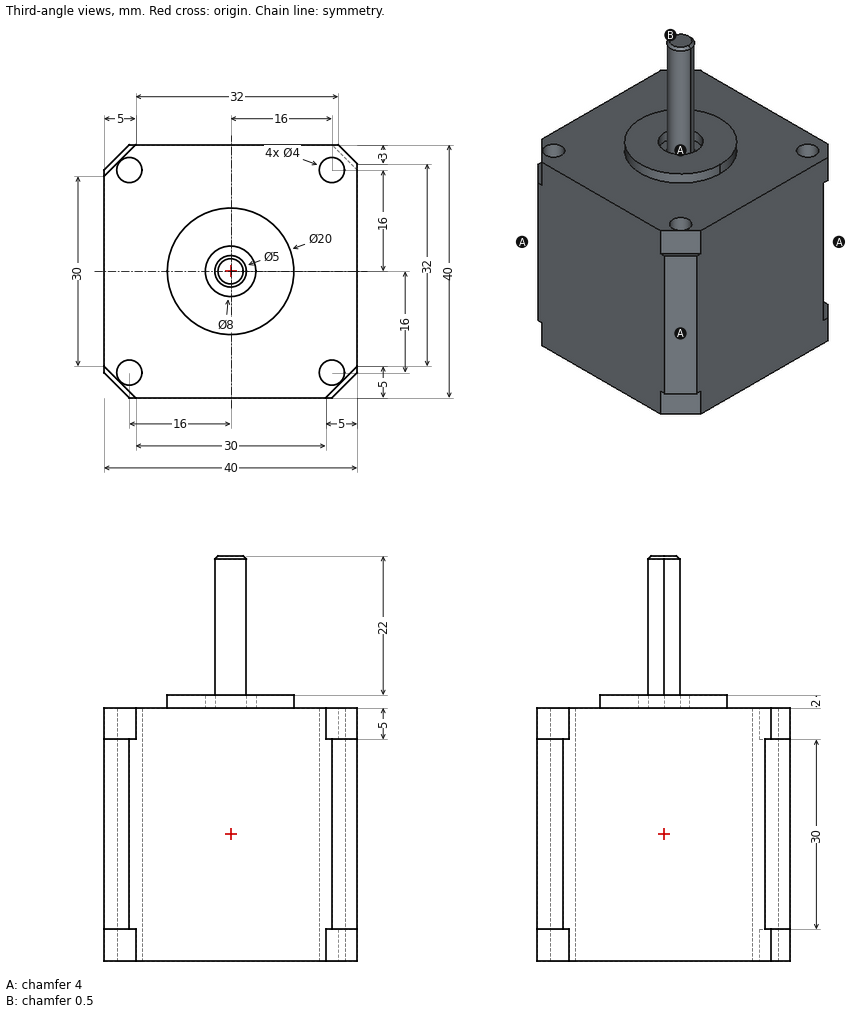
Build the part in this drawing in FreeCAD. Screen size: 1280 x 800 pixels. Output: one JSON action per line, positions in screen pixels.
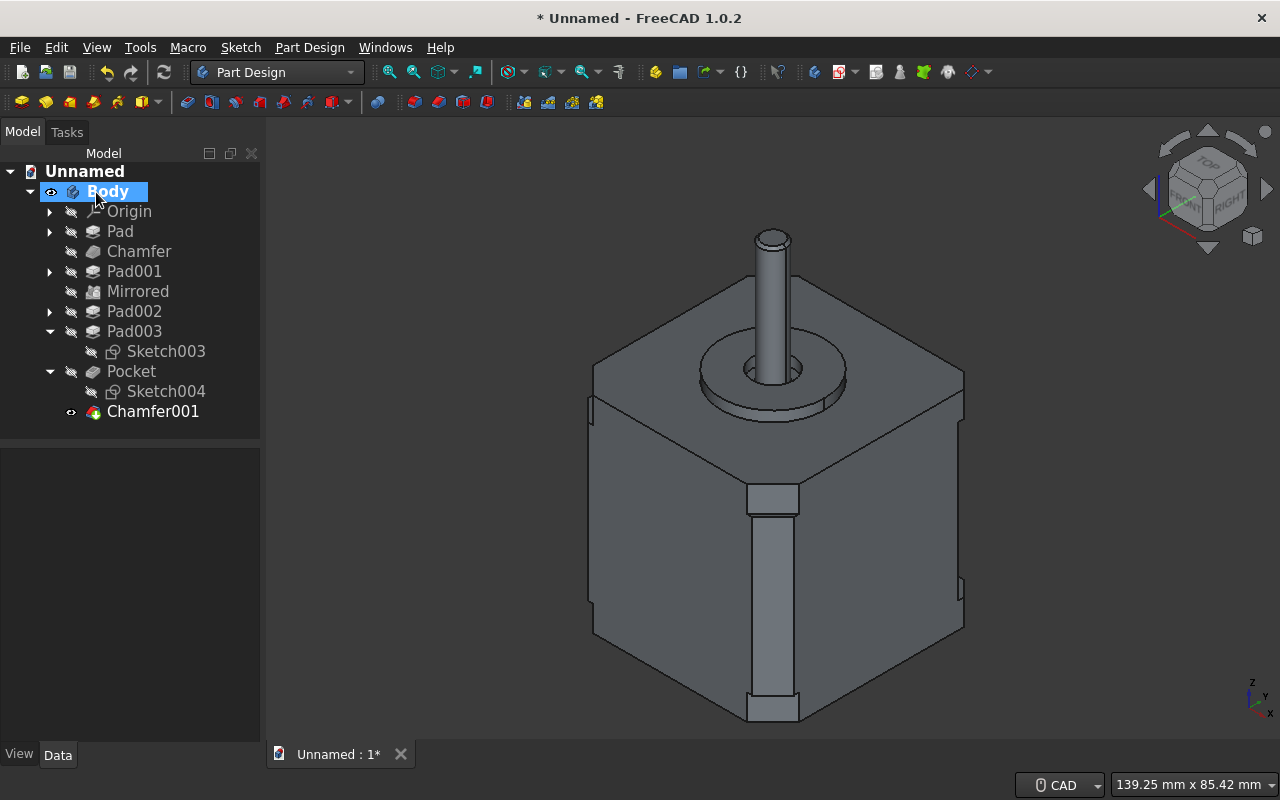
{"action": "left_click", "coordinate": [655, 379]}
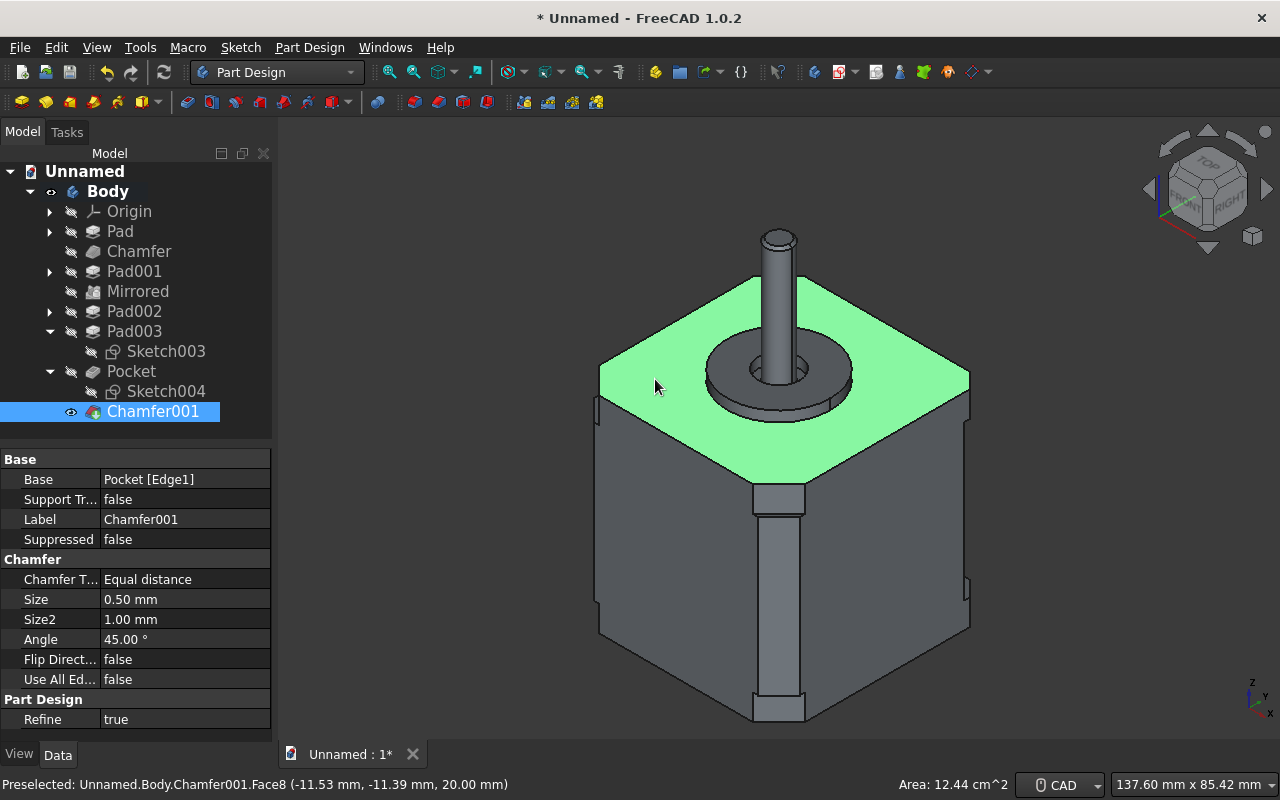
{"action": "left_click", "coordinate": [840, 72]}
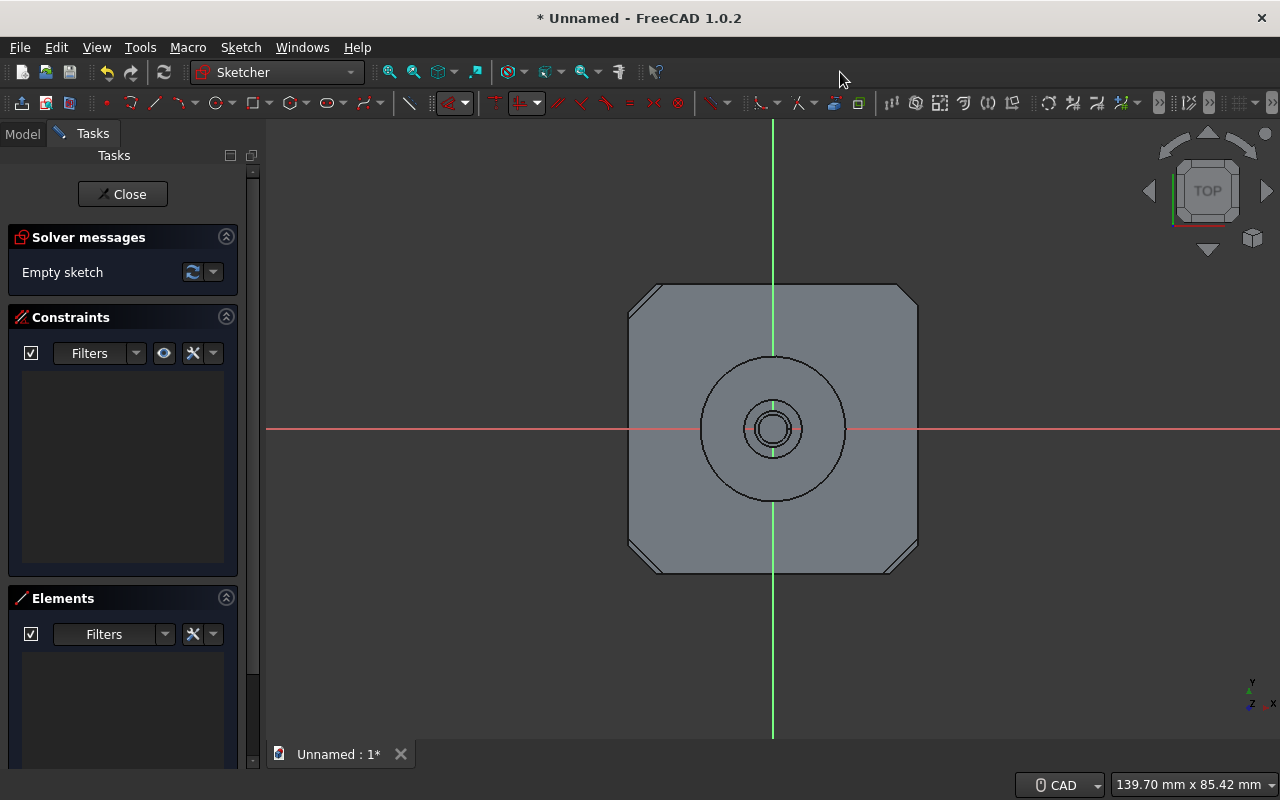
{"action": "key", "text": "q s"}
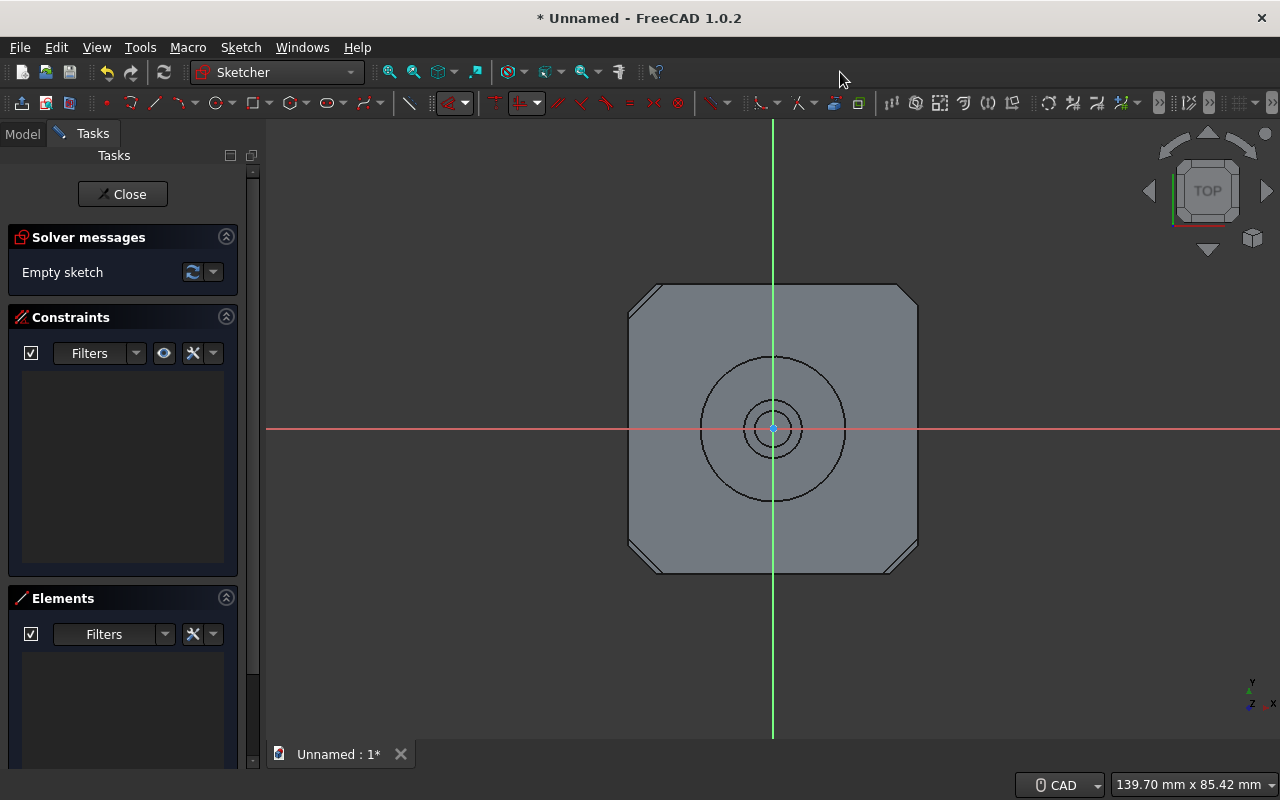
{"action": "scroll", "coordinate": [912, 429], "scroll_direction": "up", "scroll_amount": 2}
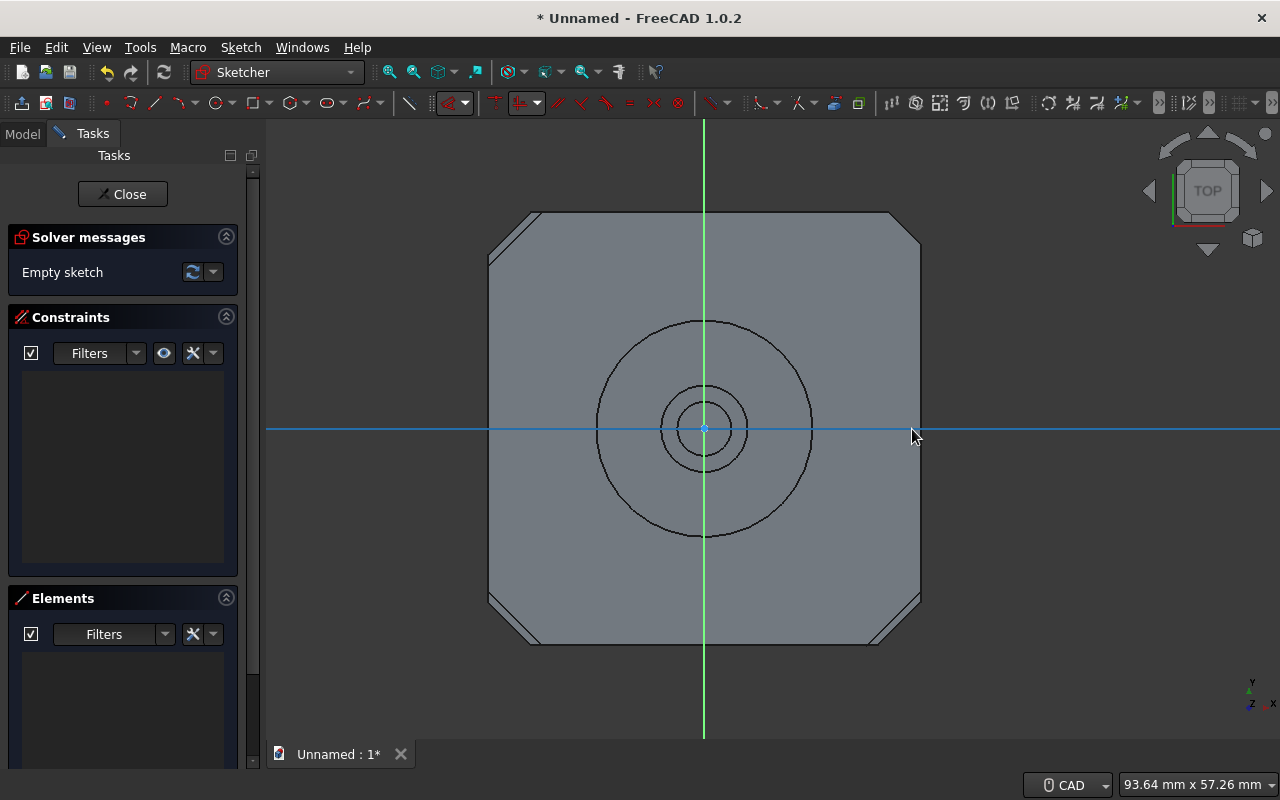
{"action": "key", "text": "g c"}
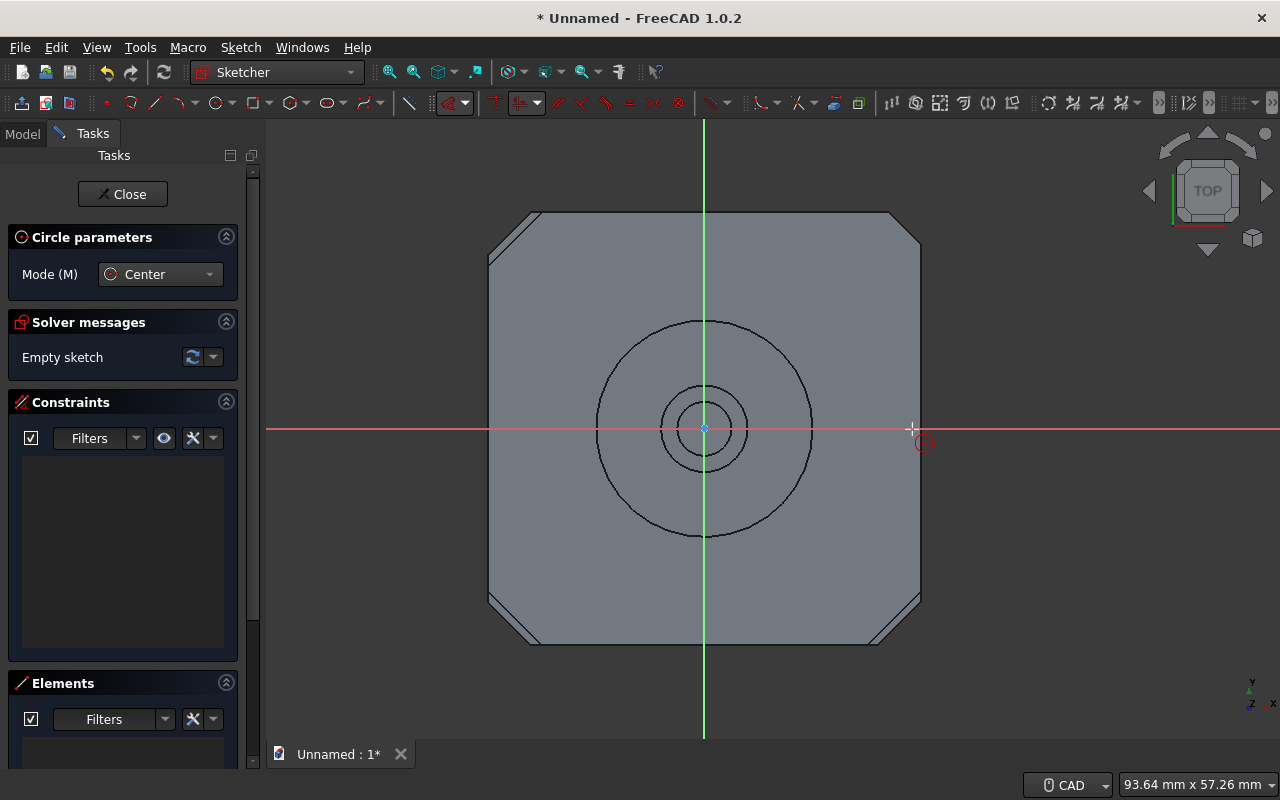
{"action": "left_click", "coordinate": [878, 255]}
{"action": "mouse_move", "coordinate": [893, 240]}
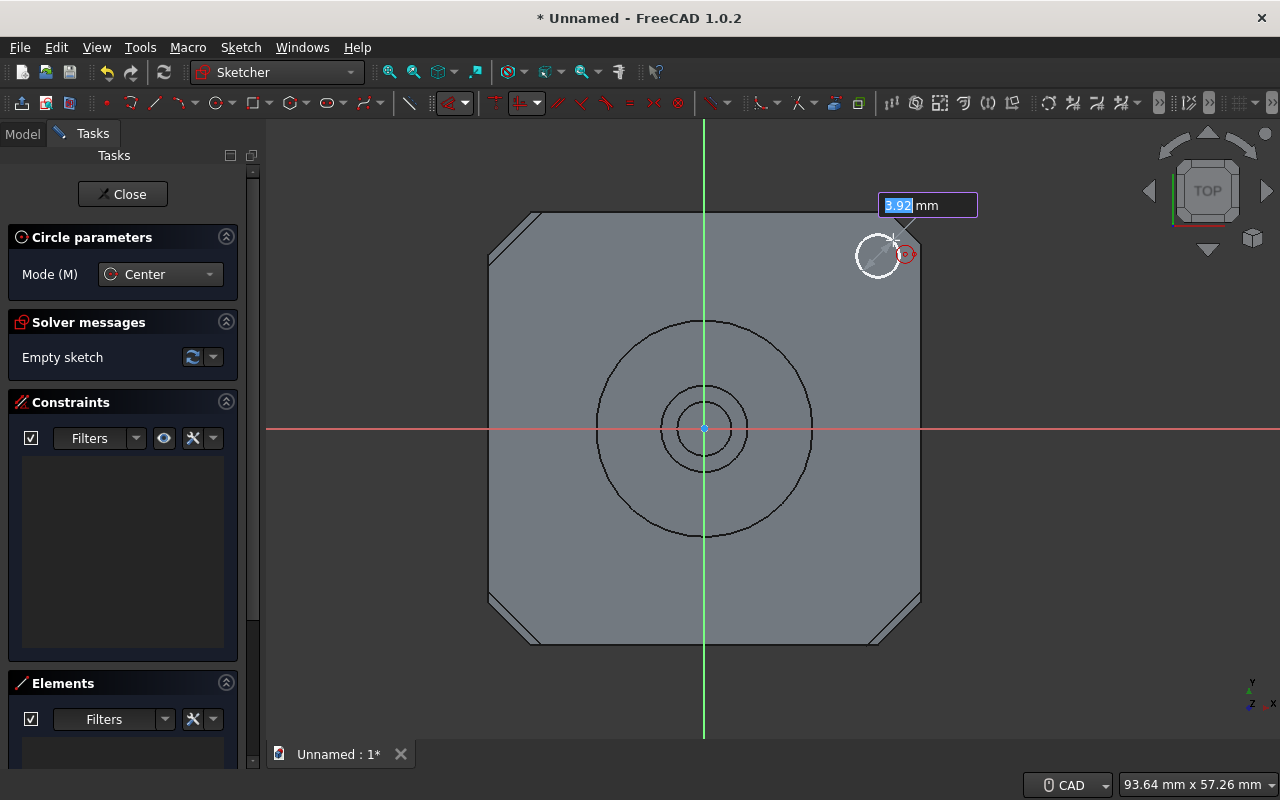
{"action": "type", "text": "4"}
{"action": "key", "text": "Return"}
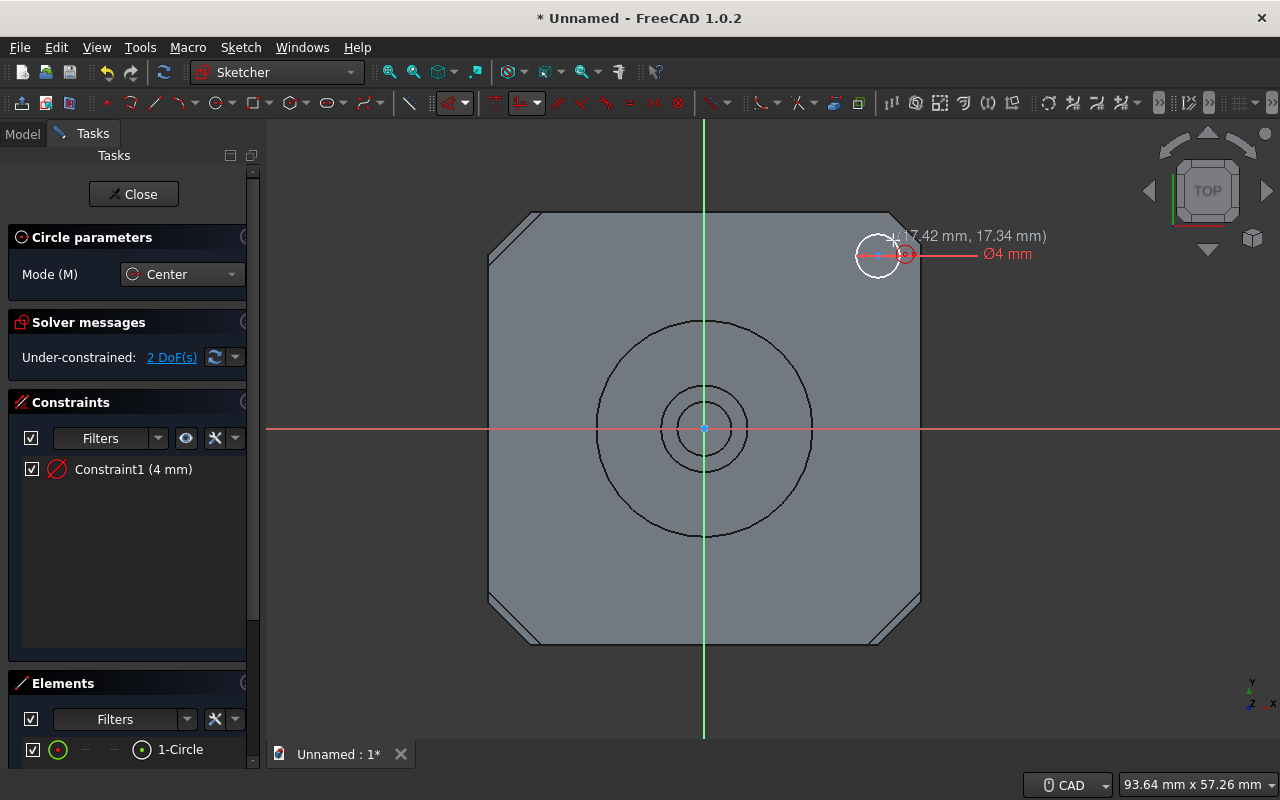
{"action": "left_click", "coordinate": [878, 602]}
{"action": "mouse_move", "coordinate": [893, 587]}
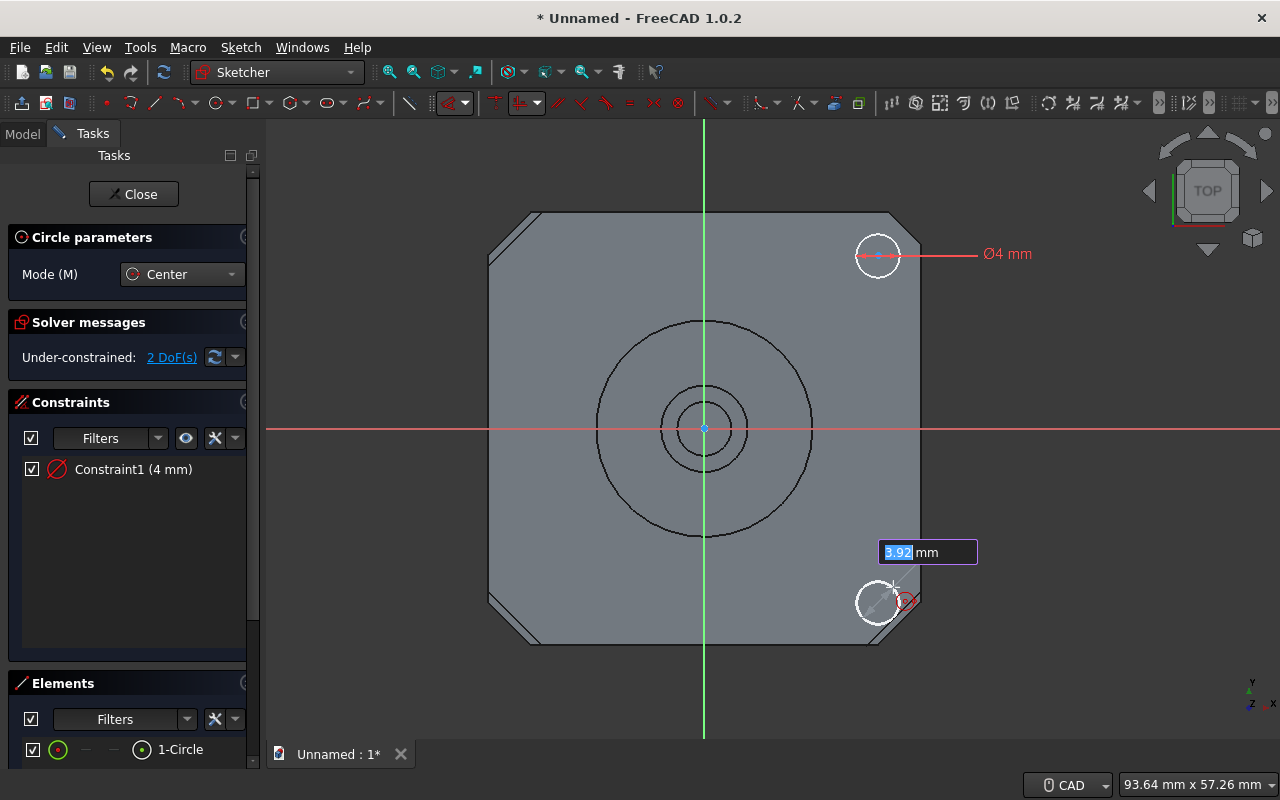
{"action": "type", "text": "4"}
{"action": "key", "text": "Return"}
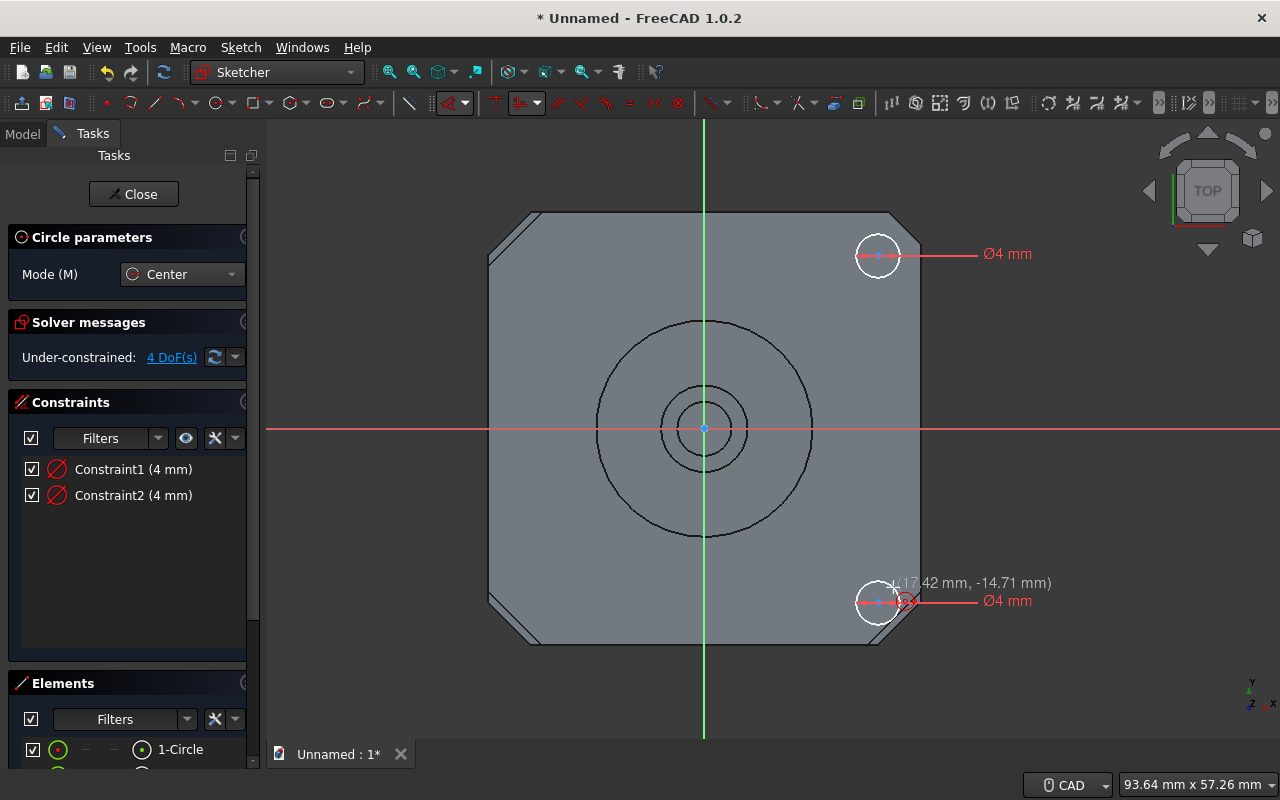
{"action": "left_click", "coordinate": [531, 602]}
{"action": "mouse_move", "coordinate": [546, 587]}